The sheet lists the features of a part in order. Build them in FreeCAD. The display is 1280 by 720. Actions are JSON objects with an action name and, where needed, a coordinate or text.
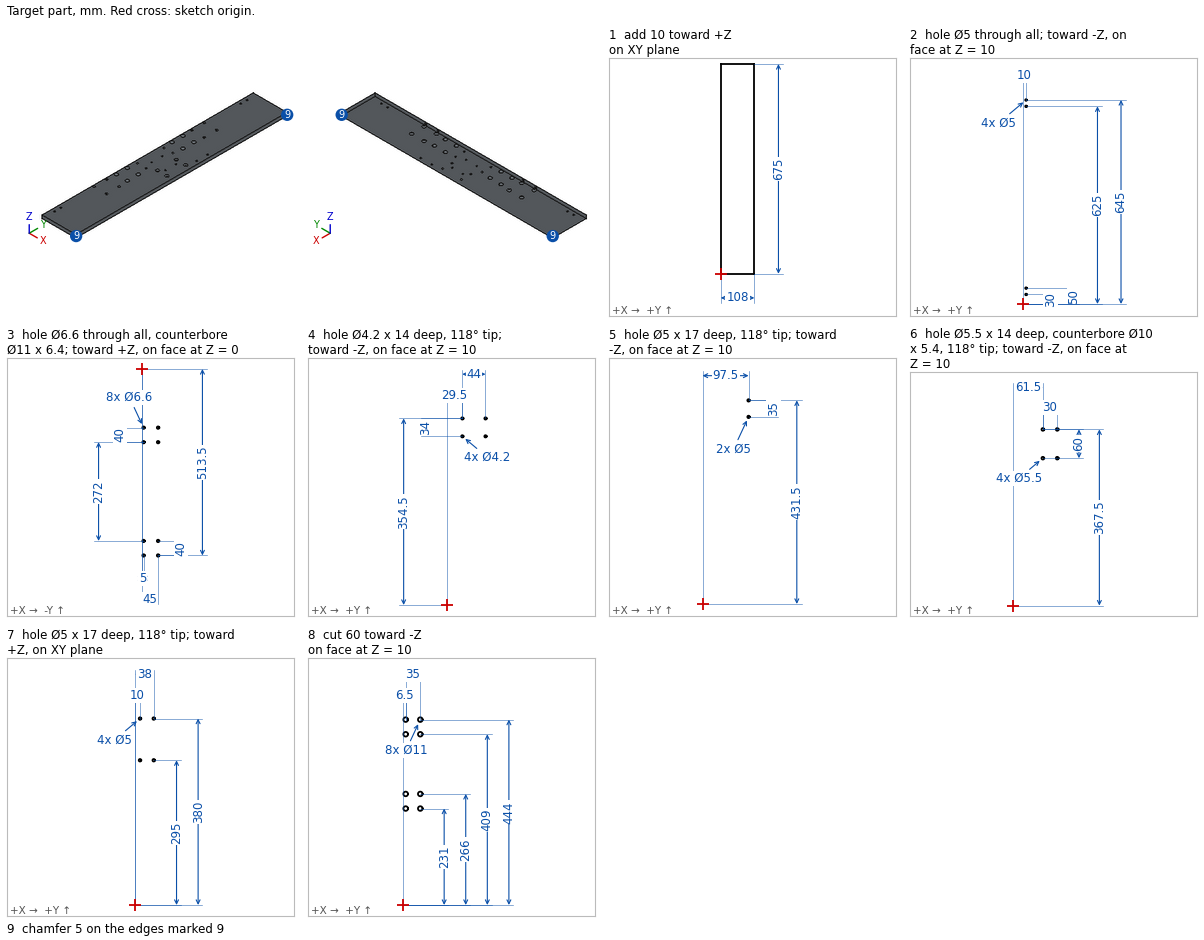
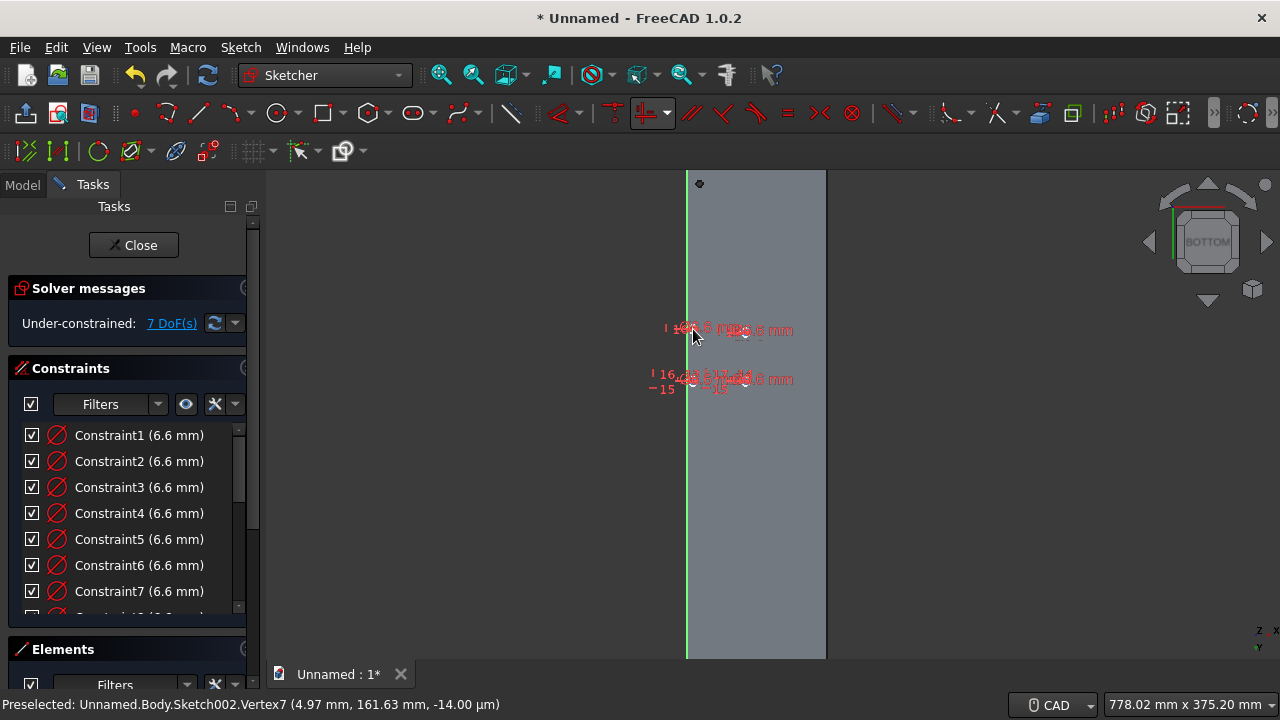
{"action": "left_click", "coordinate": [746, 333]}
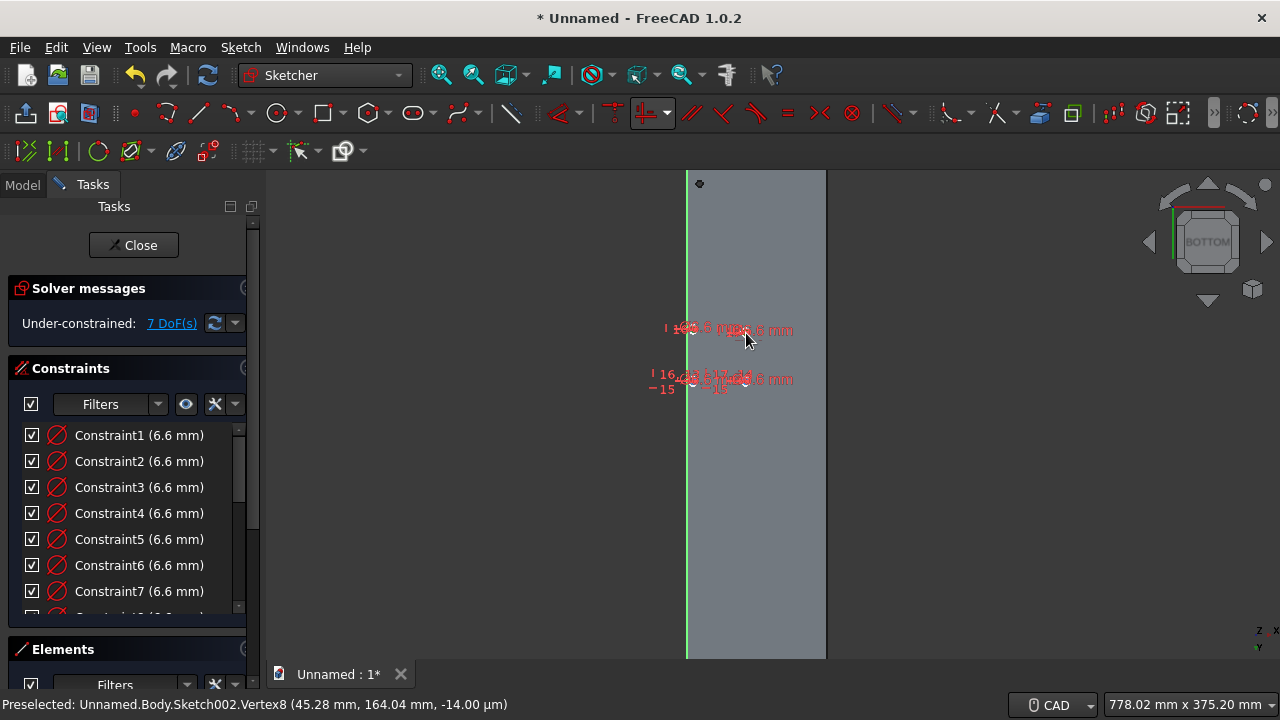
{"action": "key", "text": "h"}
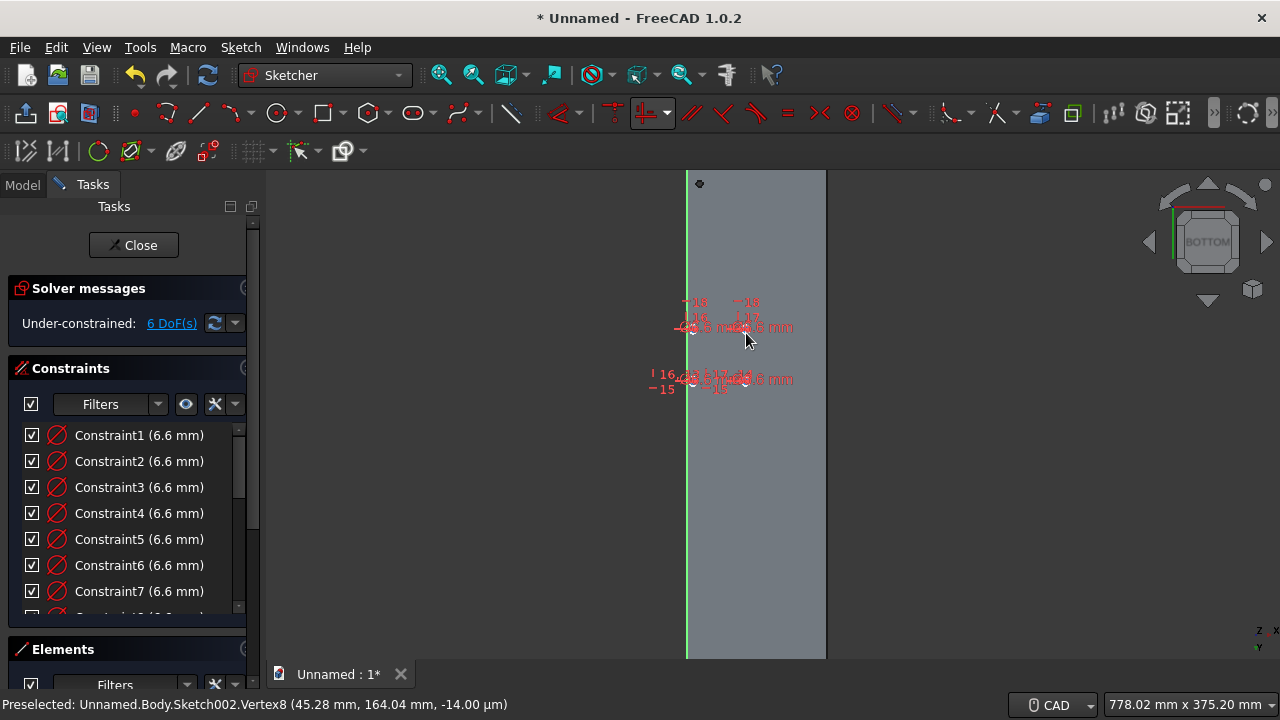
{"action": "left_click", "coordinate": [558, 114]}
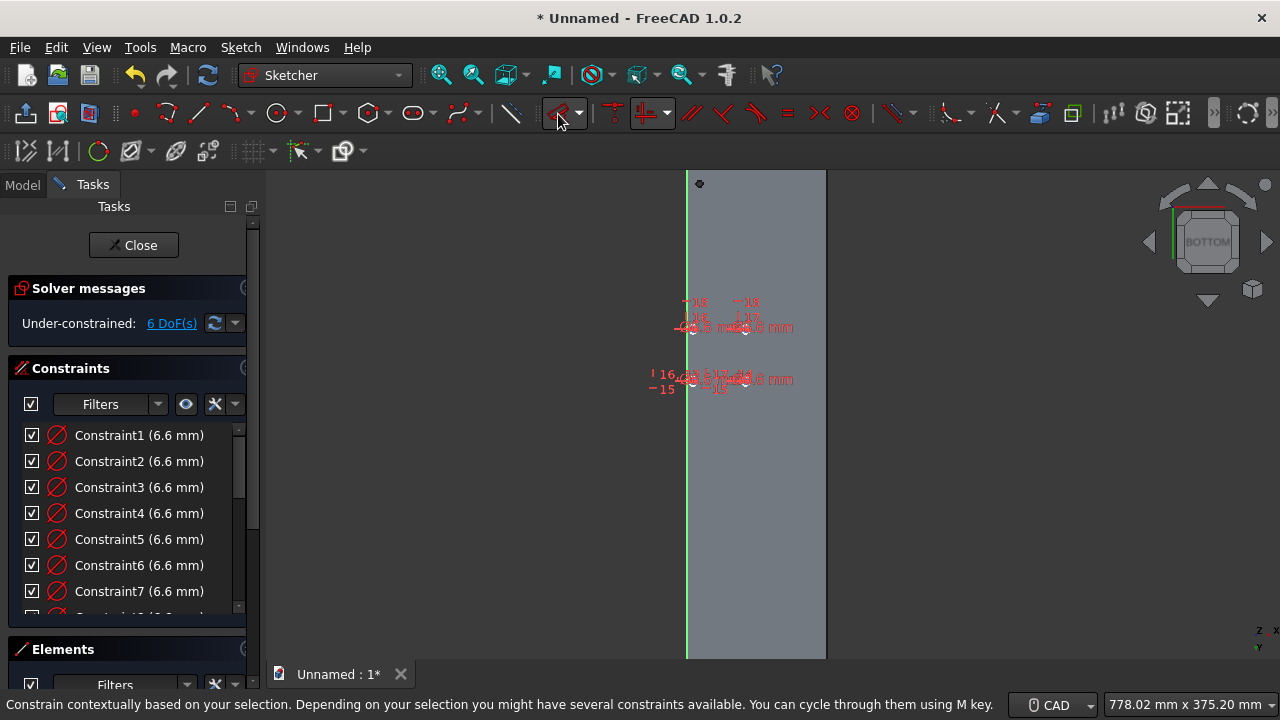
{"action": "scroll", "coordinate": [693, 381], "scroll_direction": "down", "scroll_amount": 4}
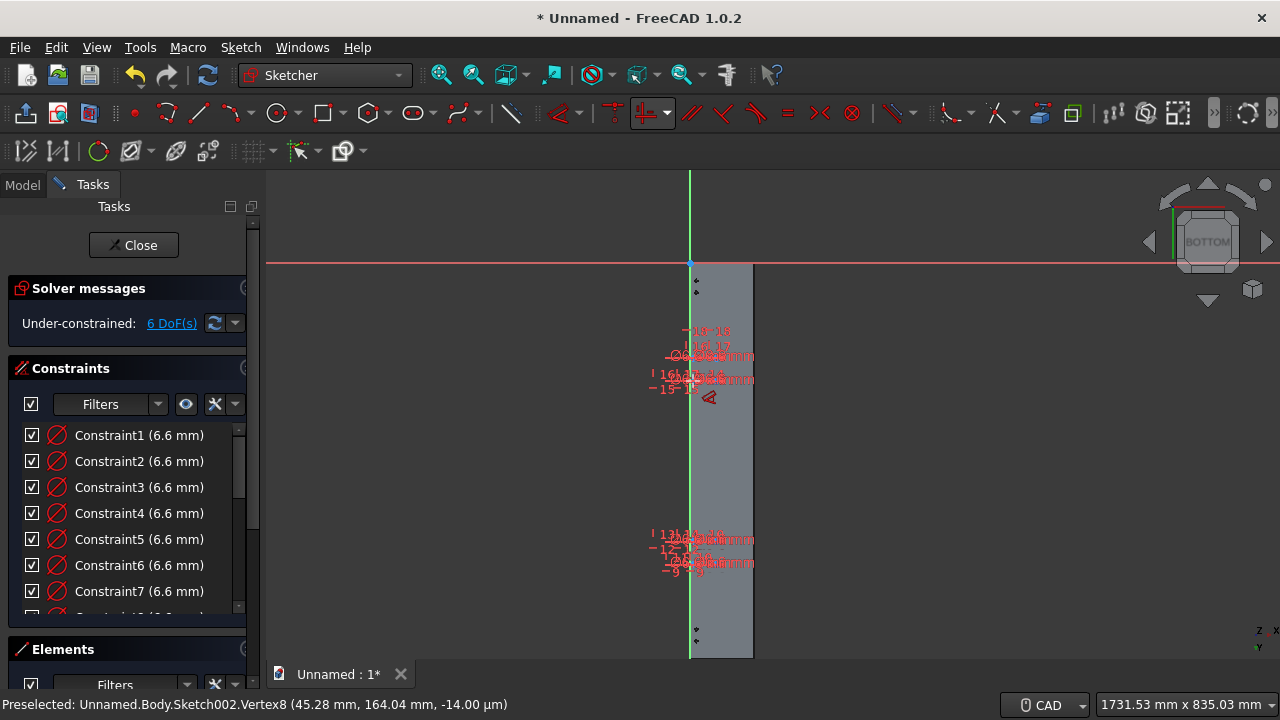
{"action": "scroll", "coordinate": [693, 565], "scroll_direction": "up", "scroll_amount": 14}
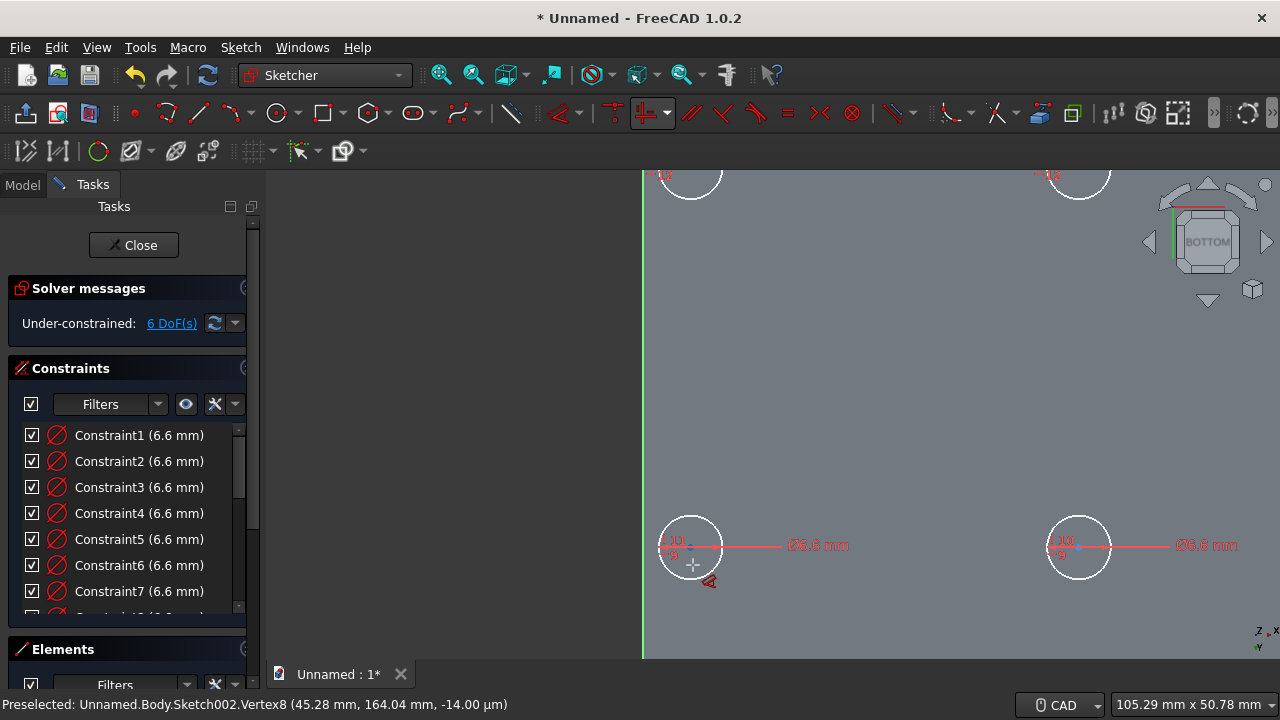
{"action": "left_click", "coordinate": [691, 547]}
{"action": "left_click", "coordinate": [667, 605]}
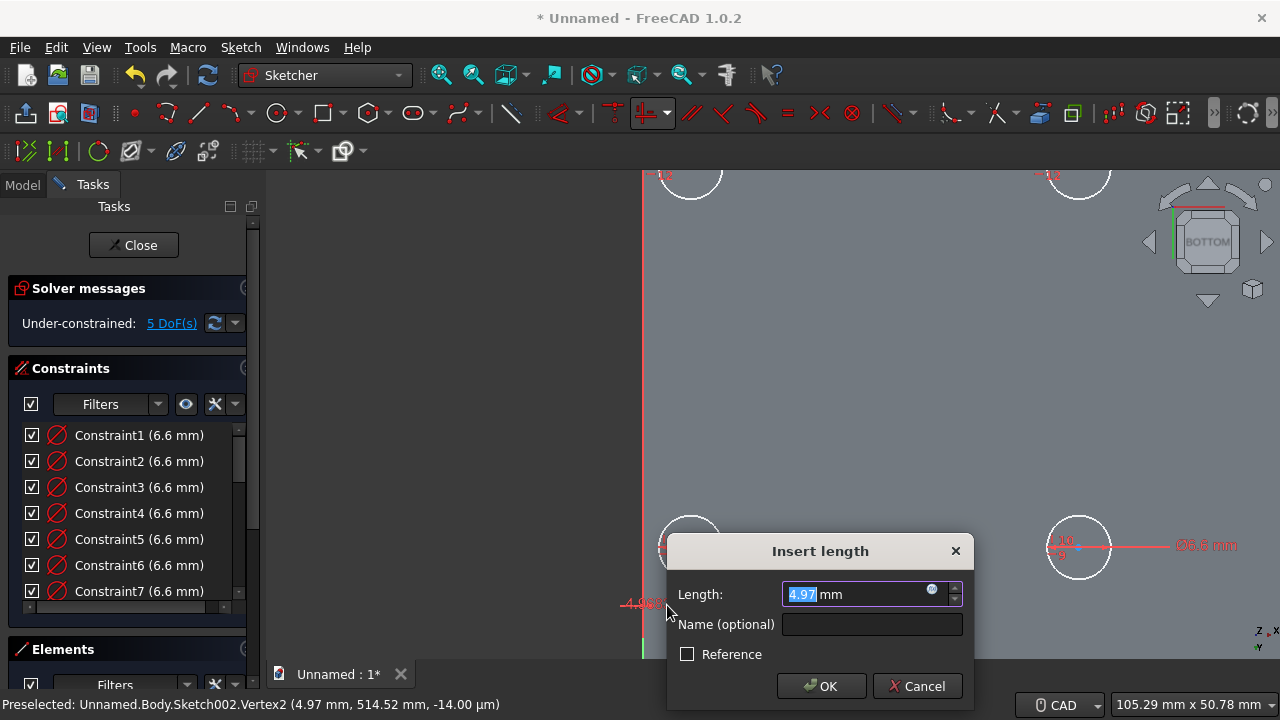
{"action": "type", "text": "5"}
{"action": "key", "text": "Return"}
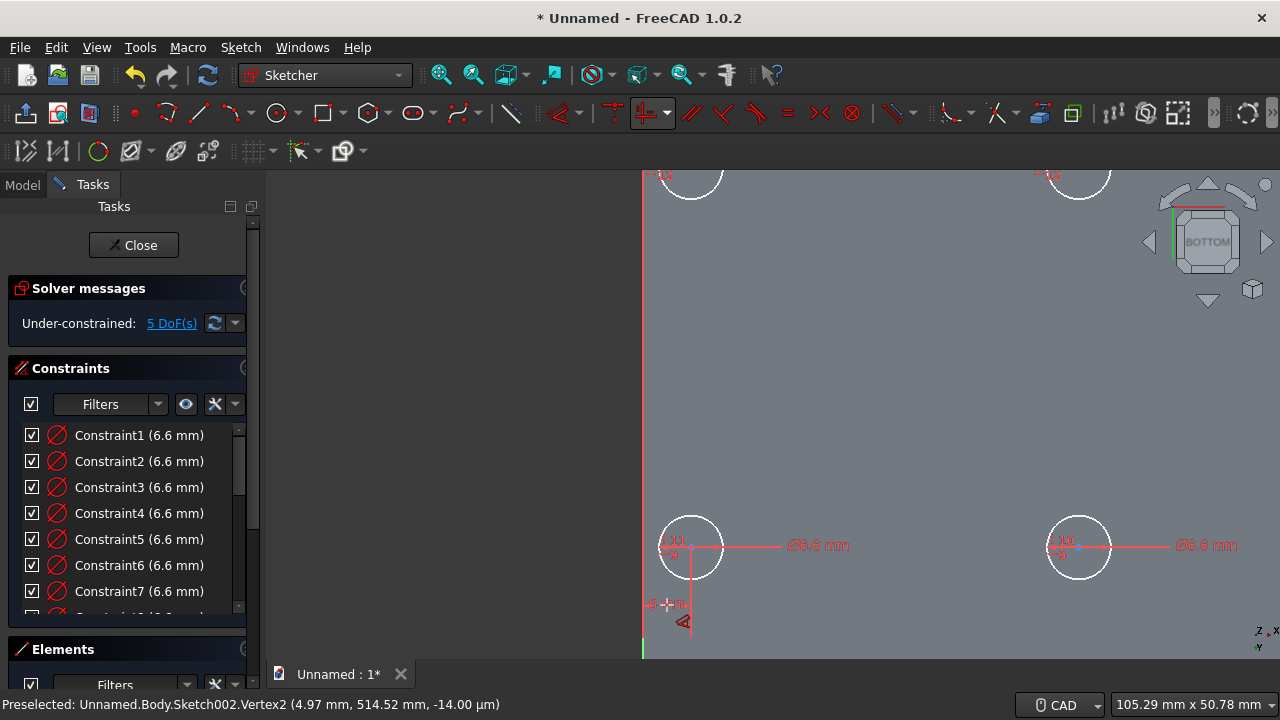
{"action": "scroll", "coordinate": [693, 566], "scroll_direction": "down", "scroll_amount": 14}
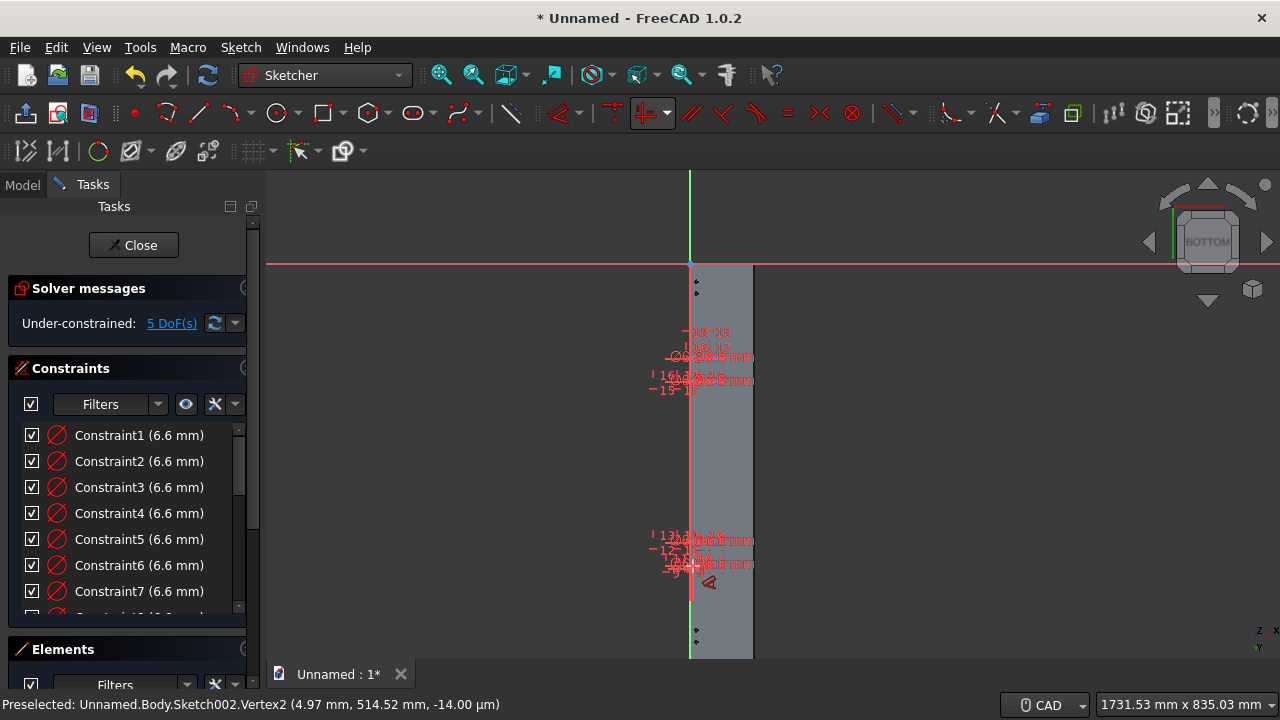
{"action": "scroll", "coordinate": [717, 566], "scroll_direction": "up", "scroll_amount": 3}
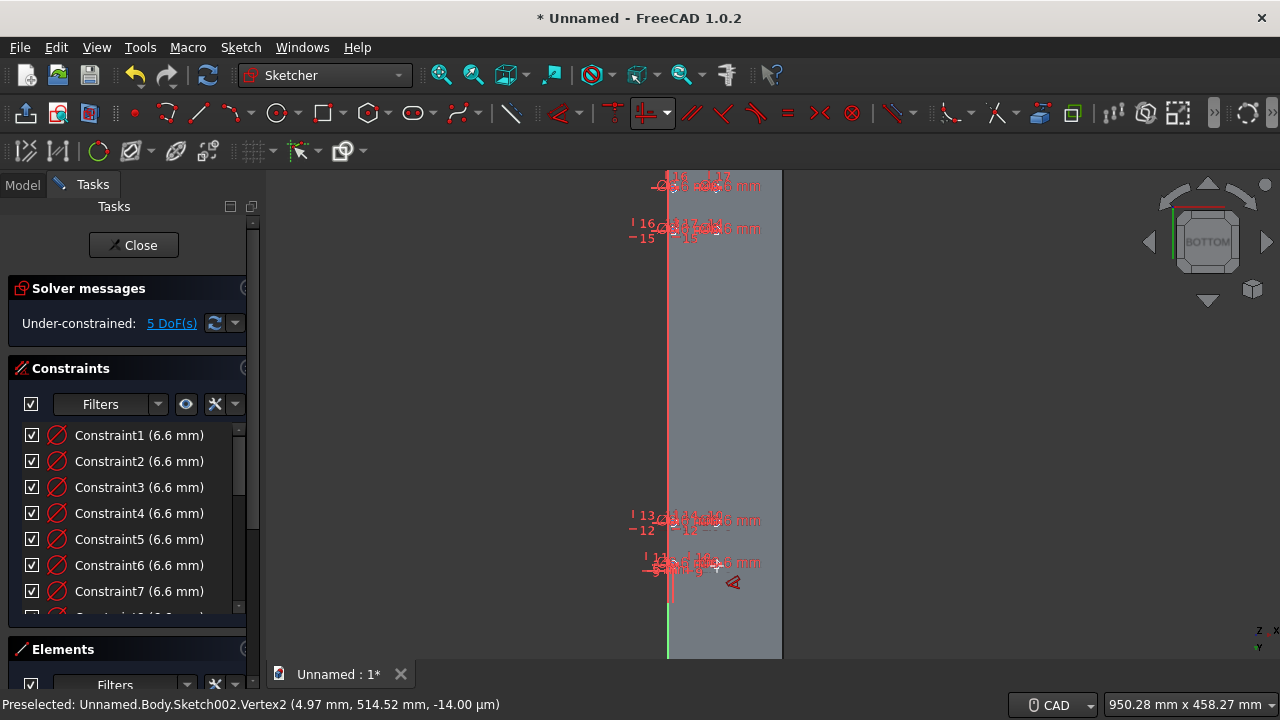
{"action": "left_click", "coordinate": [716, 565]}
{"action": "left_click", "coordinate": [692, 599]}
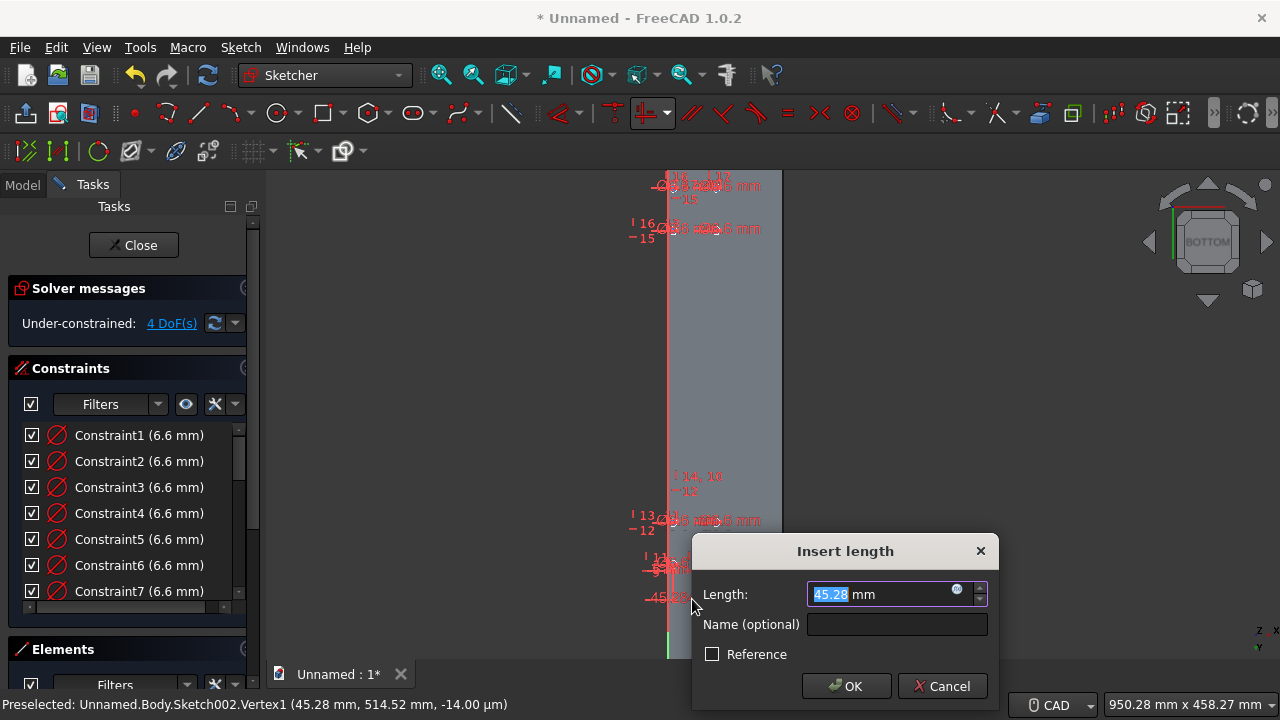
{"action": "type", "text": "45"}
{"action": "key", "text": "Return"}